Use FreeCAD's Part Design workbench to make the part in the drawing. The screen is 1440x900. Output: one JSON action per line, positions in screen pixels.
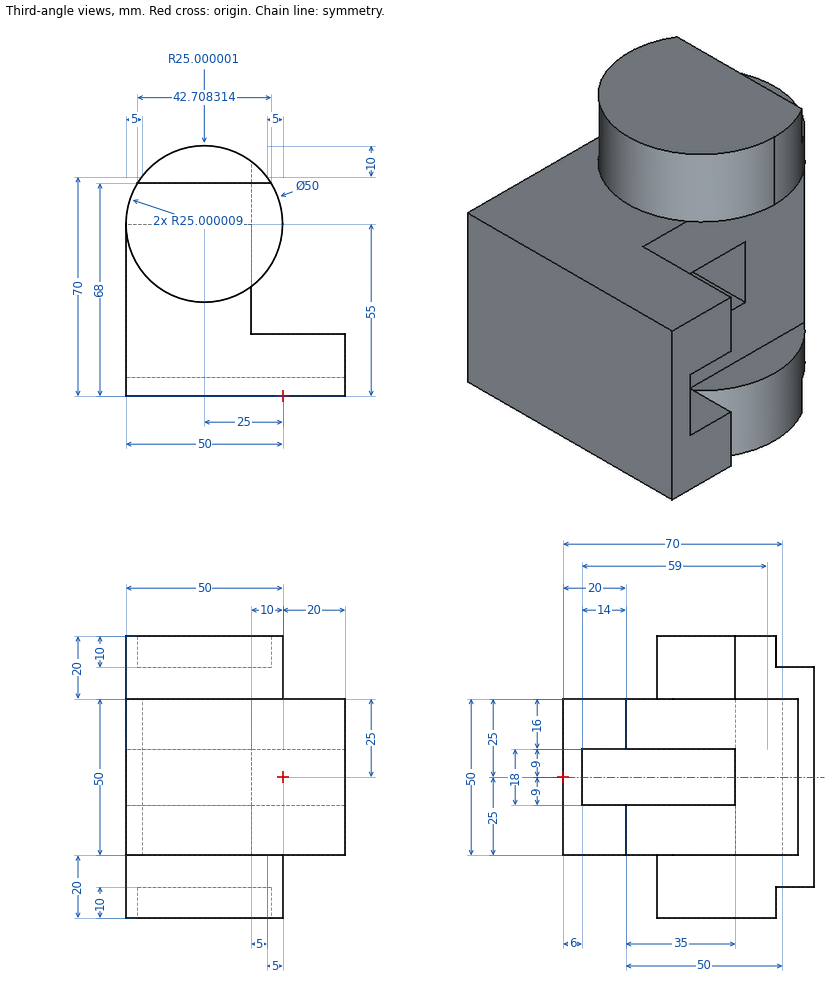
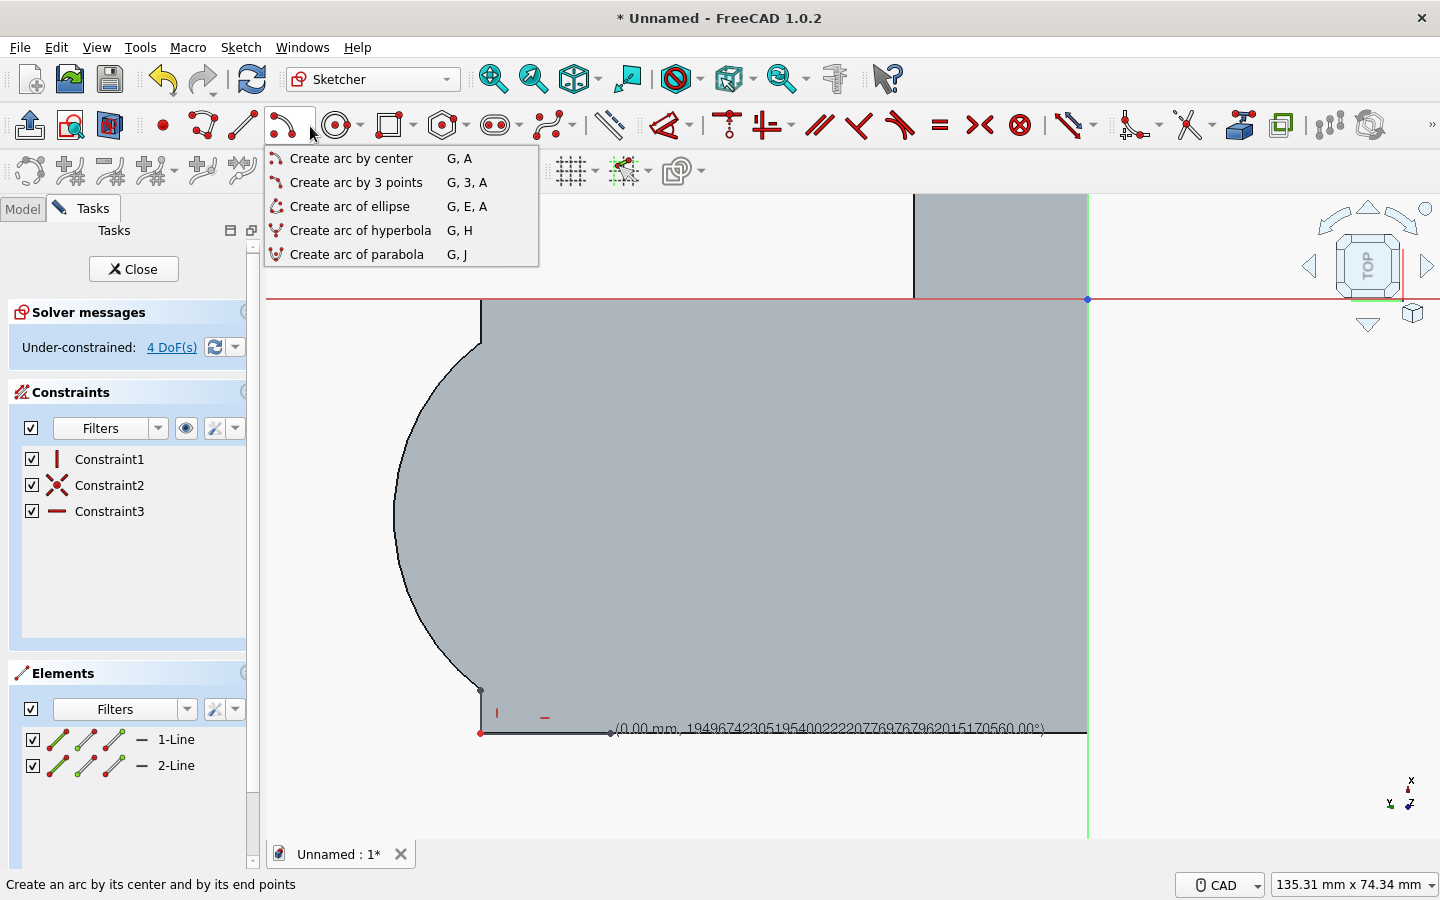
{"action": "left_click", "coordinate": [402, 182]}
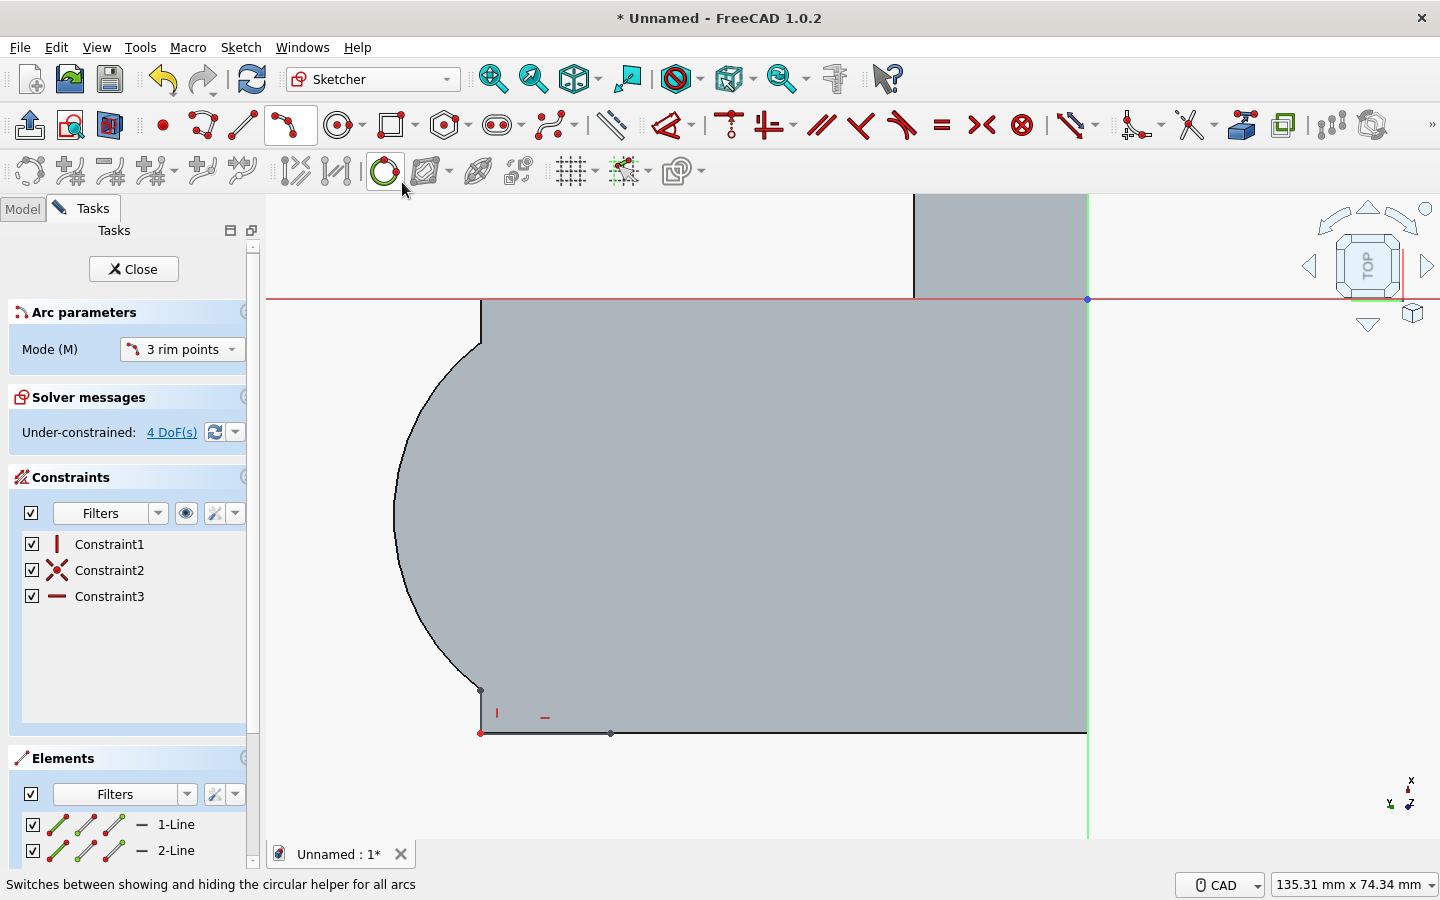
{"action": "left_click", "coordinate": [611, 734]}
{"action": "left_click", "coordinate": [481, 691]}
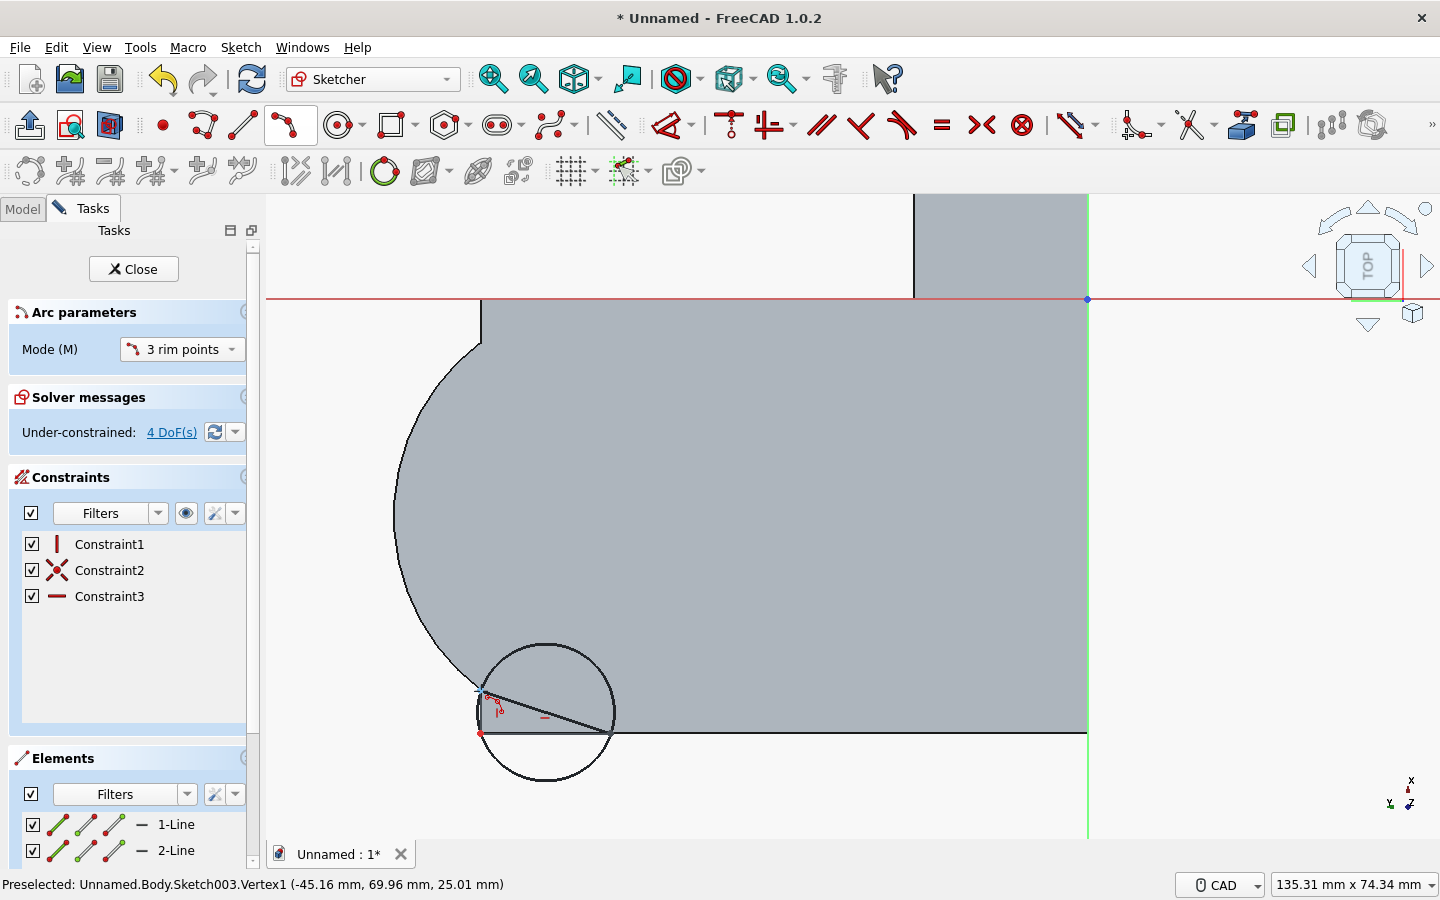
{"action": "scroll", "coordinate": [542, 722], "scroll_direction": "up", "scroll_amount": 2}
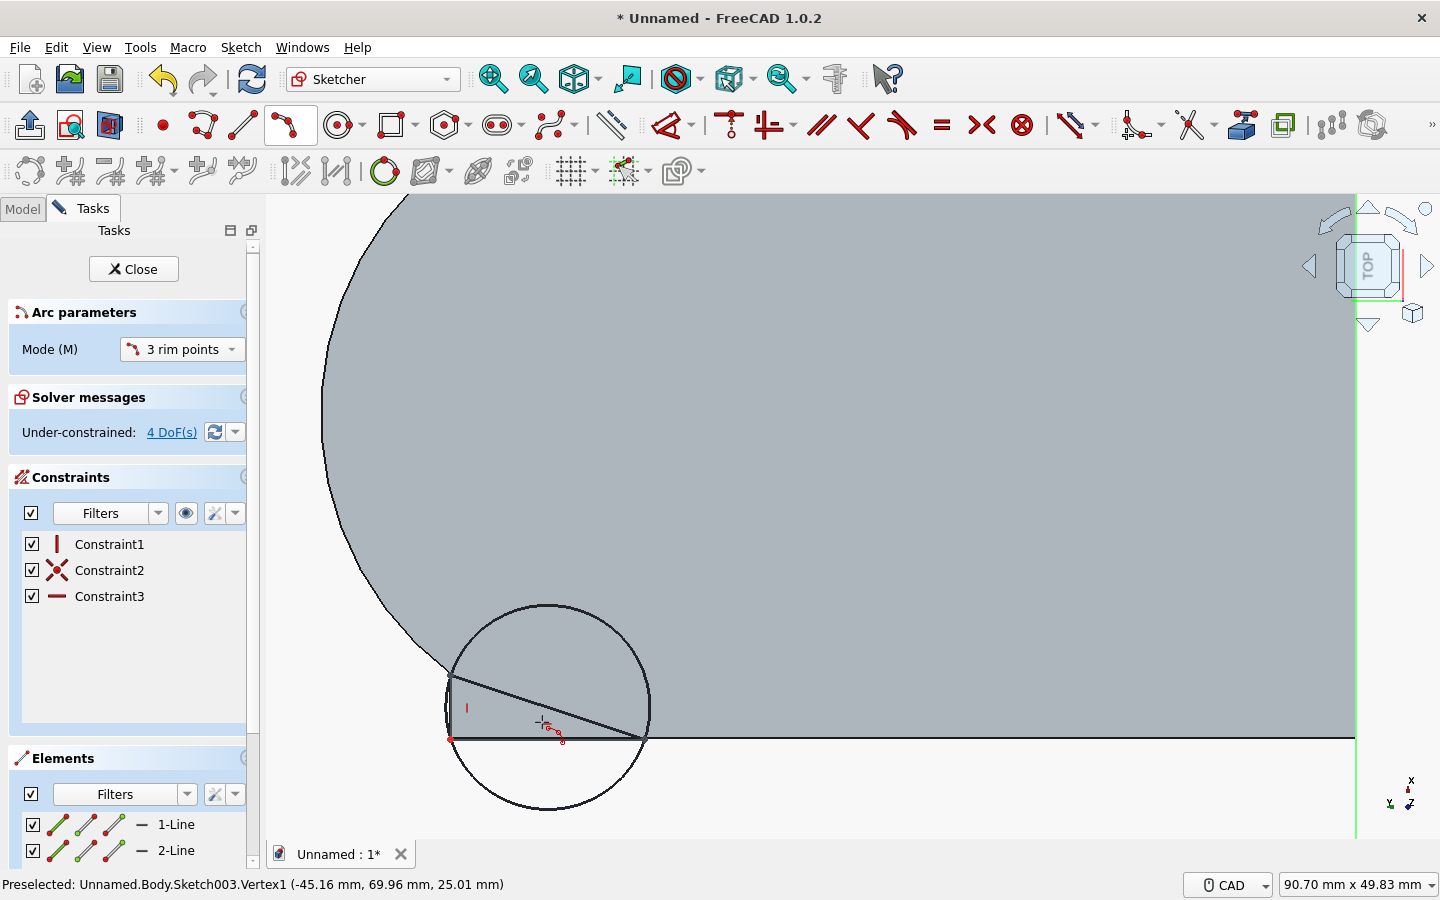
{"action": "left_click", "coordinate": [542, 721]}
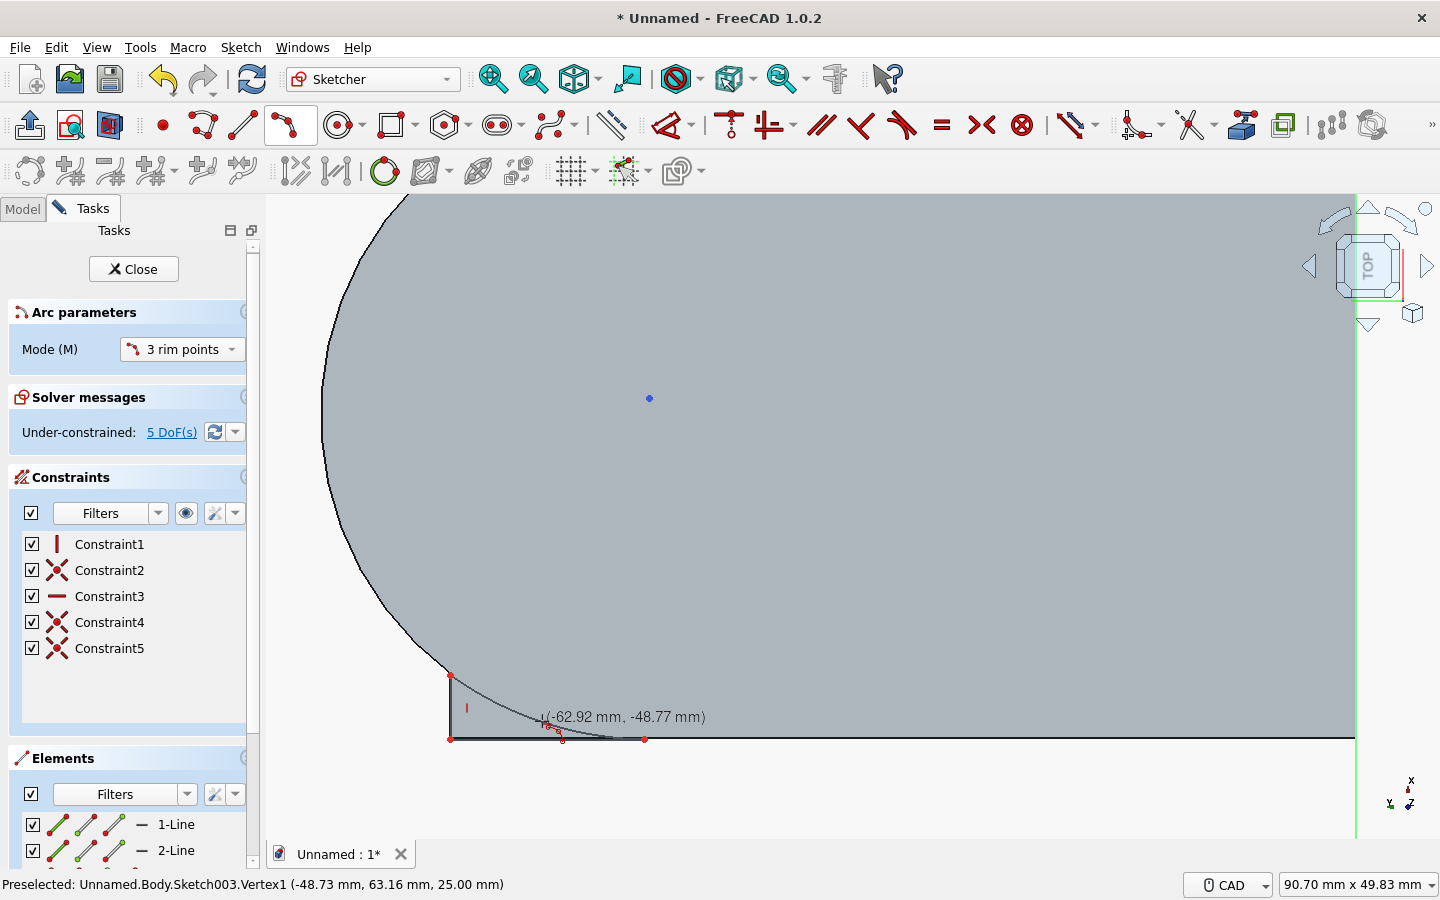
{"action": "key", "text": "g m"}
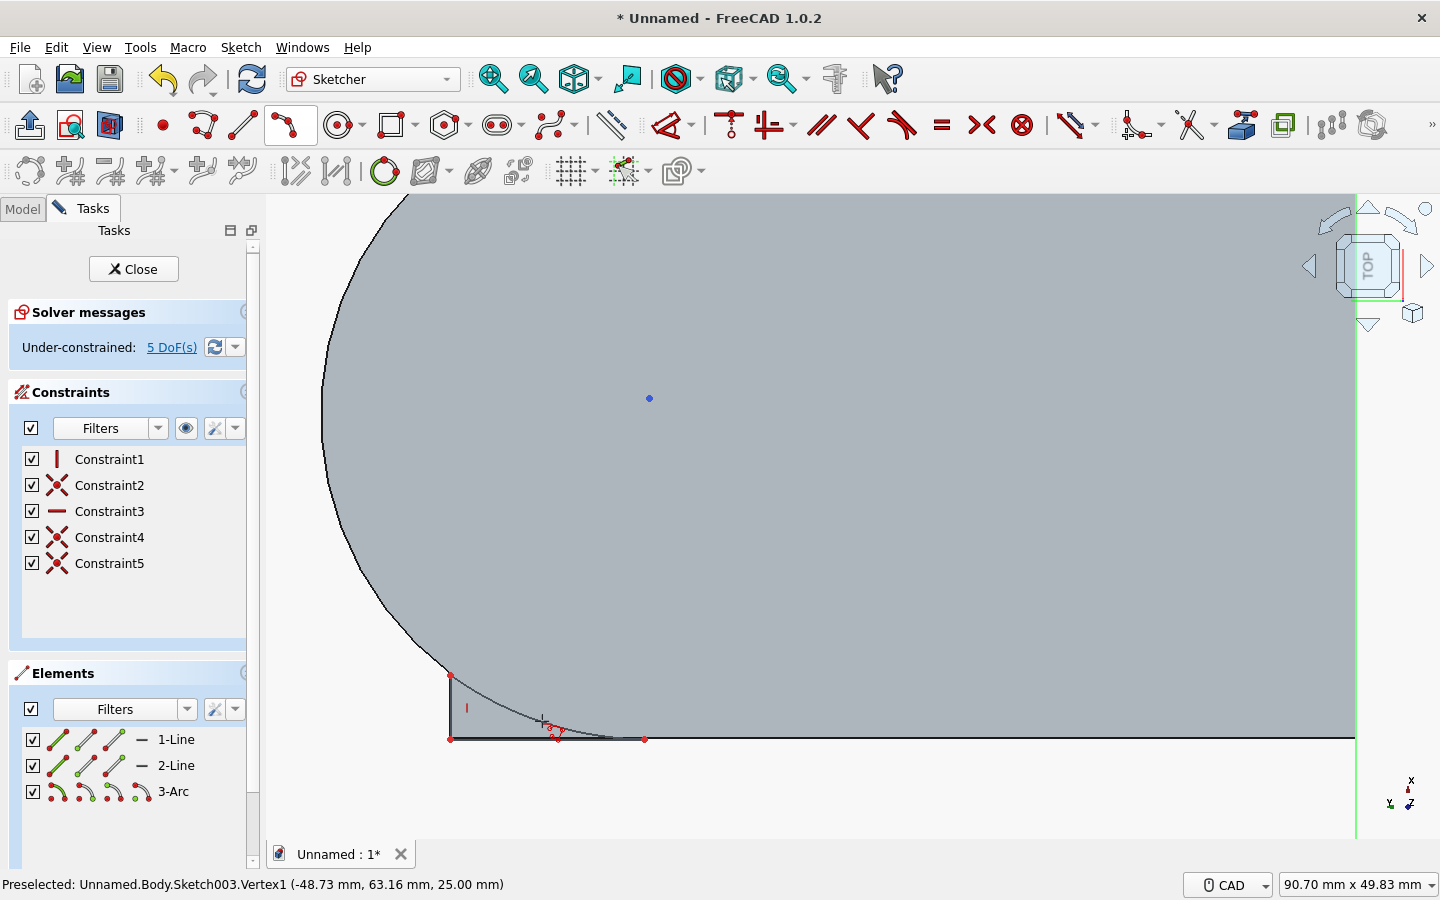
{"action": "scroll", "coordinate": [543, 724], "scroll_direction": "down", "scroll_amount": 2}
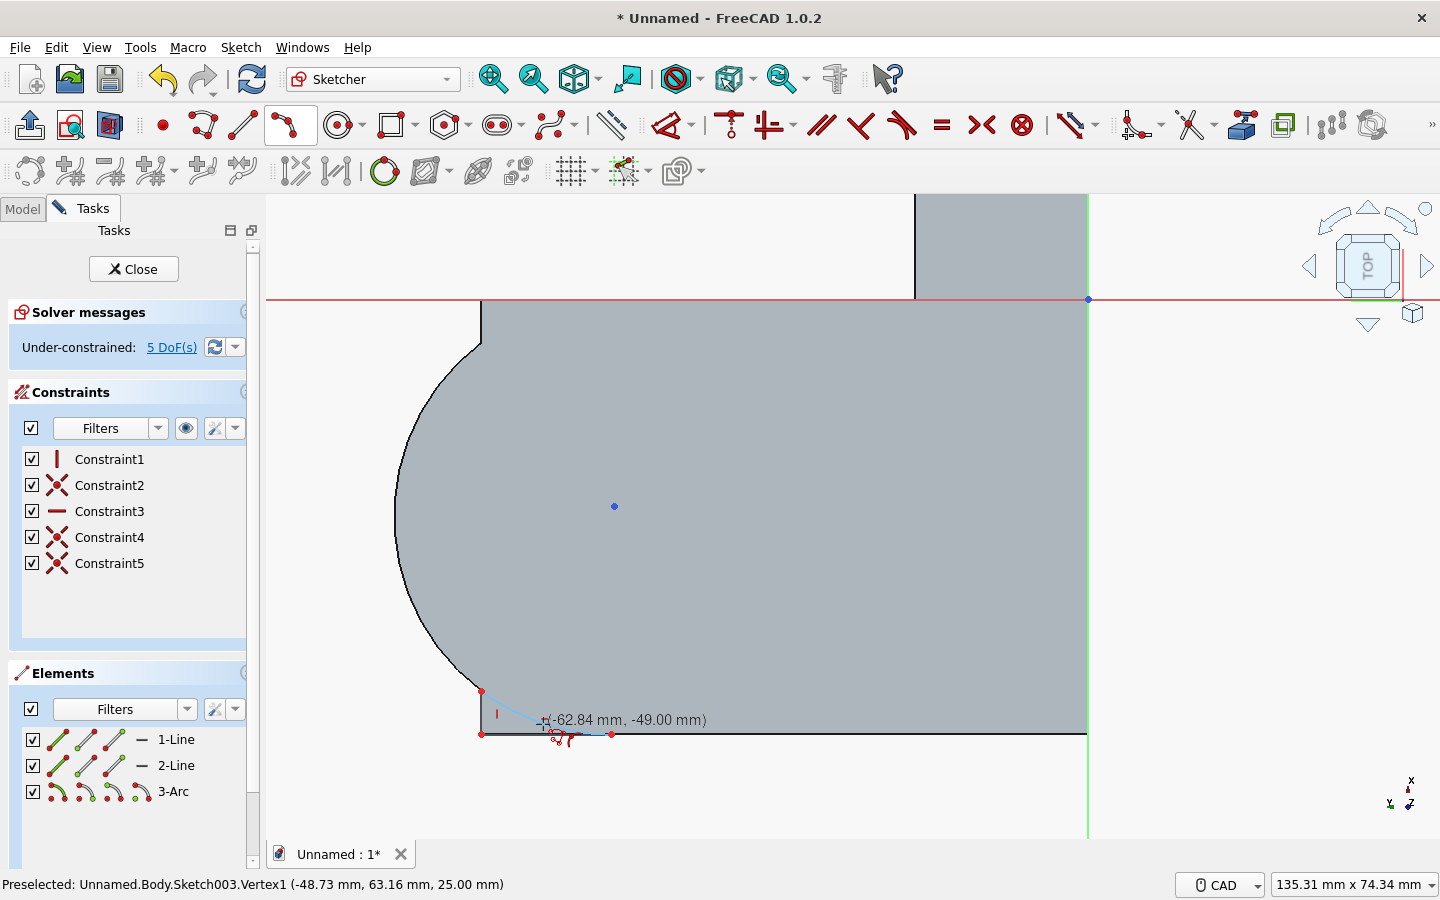
{"action": "left_click", "coordinate": [611, 300]}
{"action": "left_click", "coordinate": [481, 309]}
{"action": "left_click", "coordinate": [481, 343]}
{"action": "right_click", "coordinate": [481, 343]}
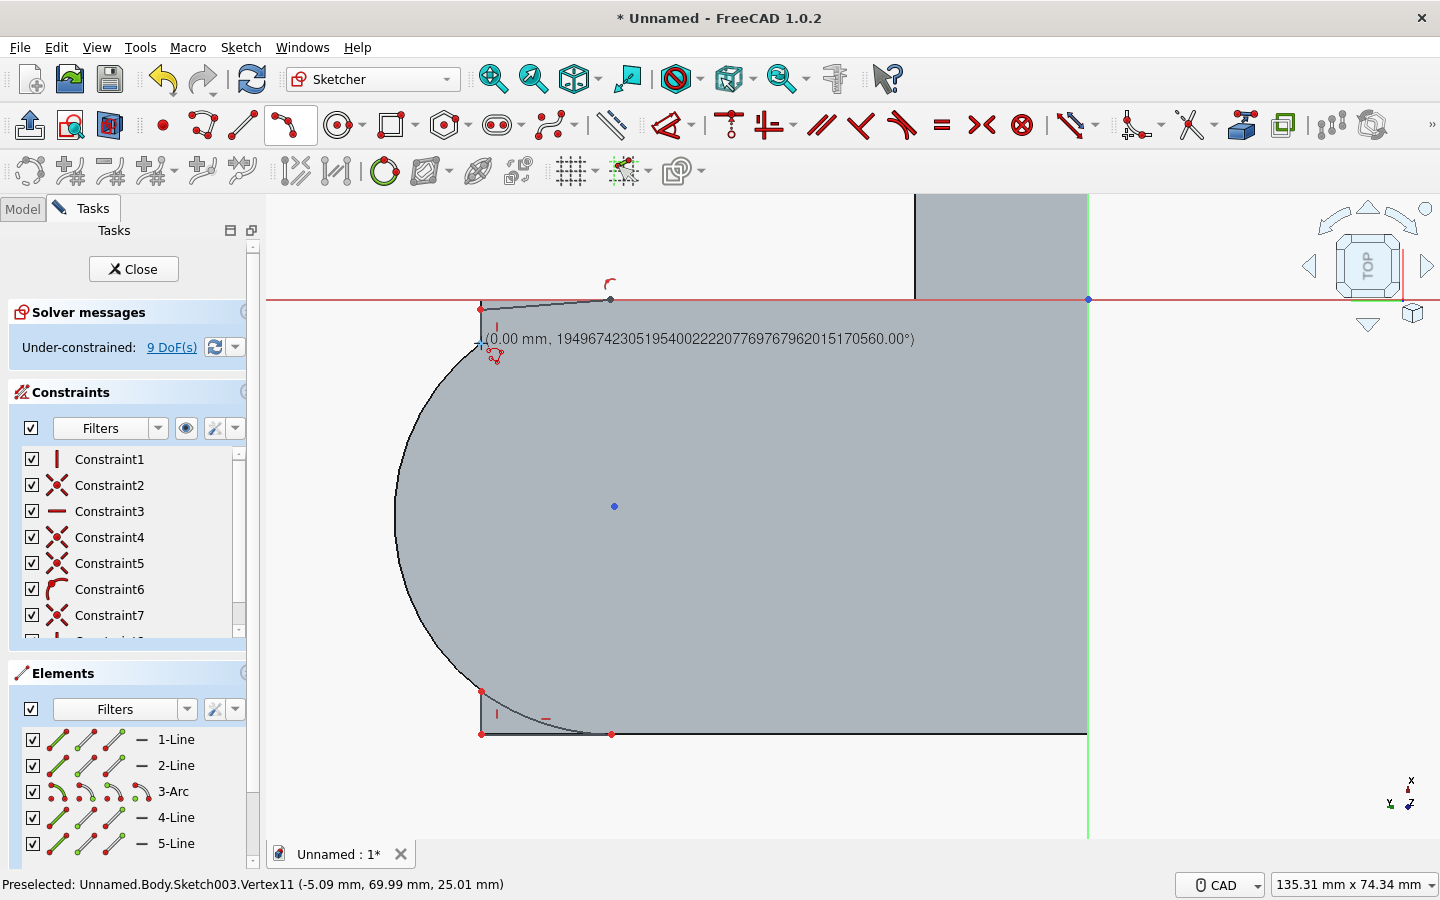
{"action": "left_click", "coordinate": [284, 126]}